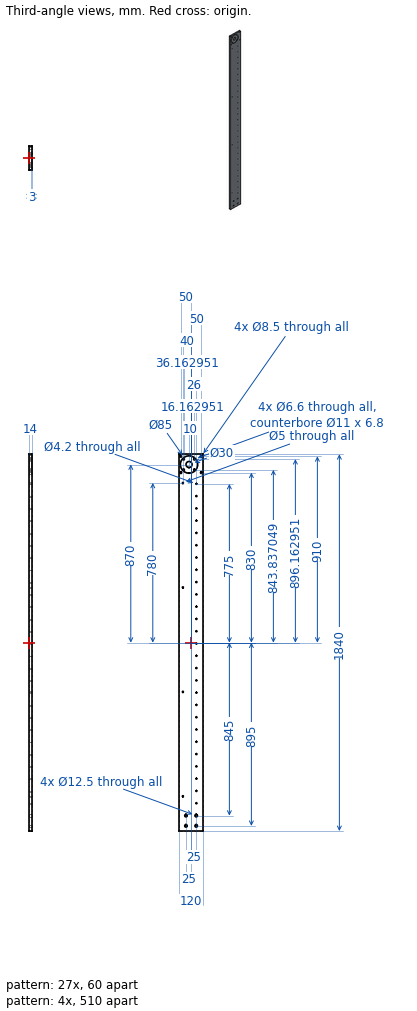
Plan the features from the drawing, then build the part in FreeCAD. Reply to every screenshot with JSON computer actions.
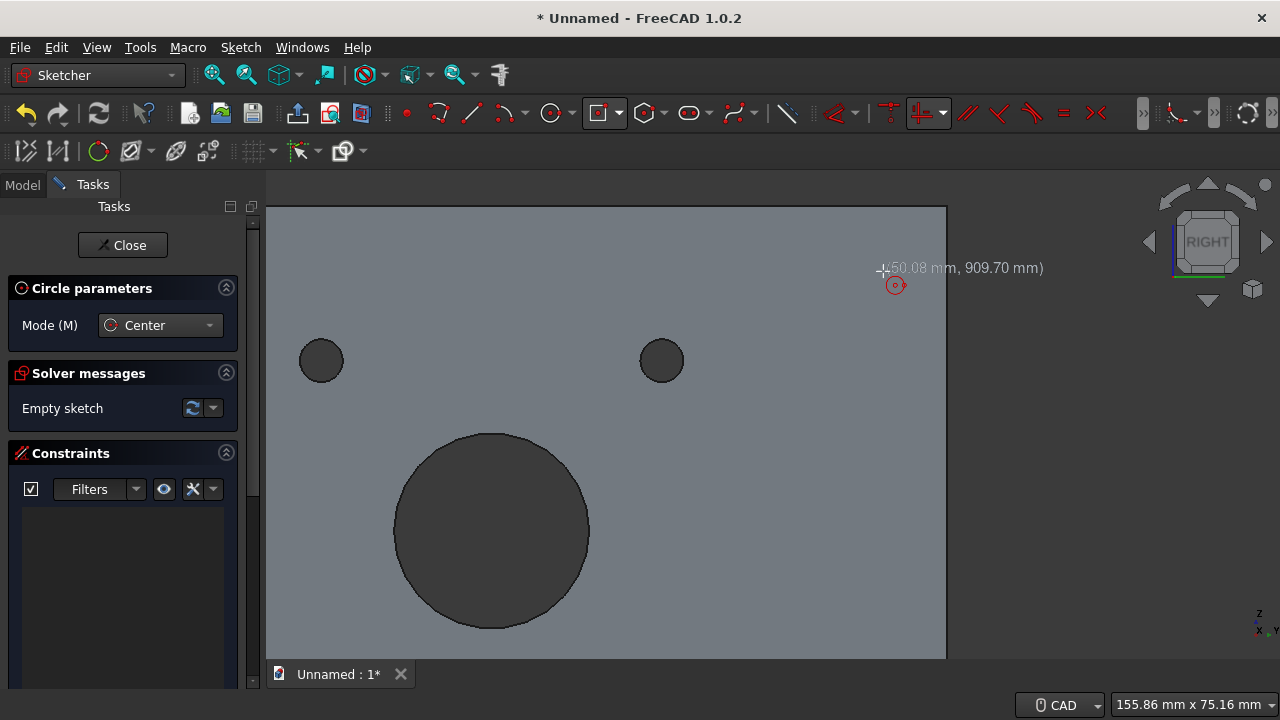
{"action": "left_click", "coordinate": [882, 271]}
{"action": "mouse_move", "coordinate": [902, 251]}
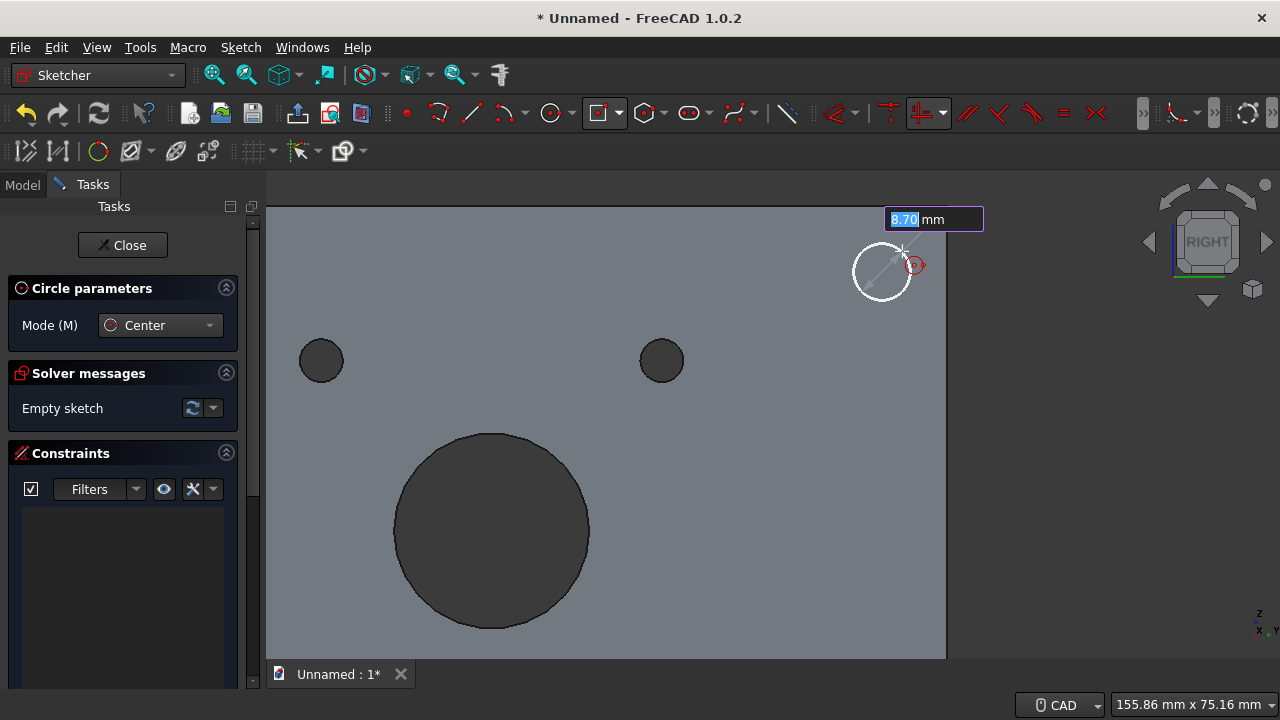
{"action": "type", "text": "8.5"}
{"action": "key", "text": "Return"}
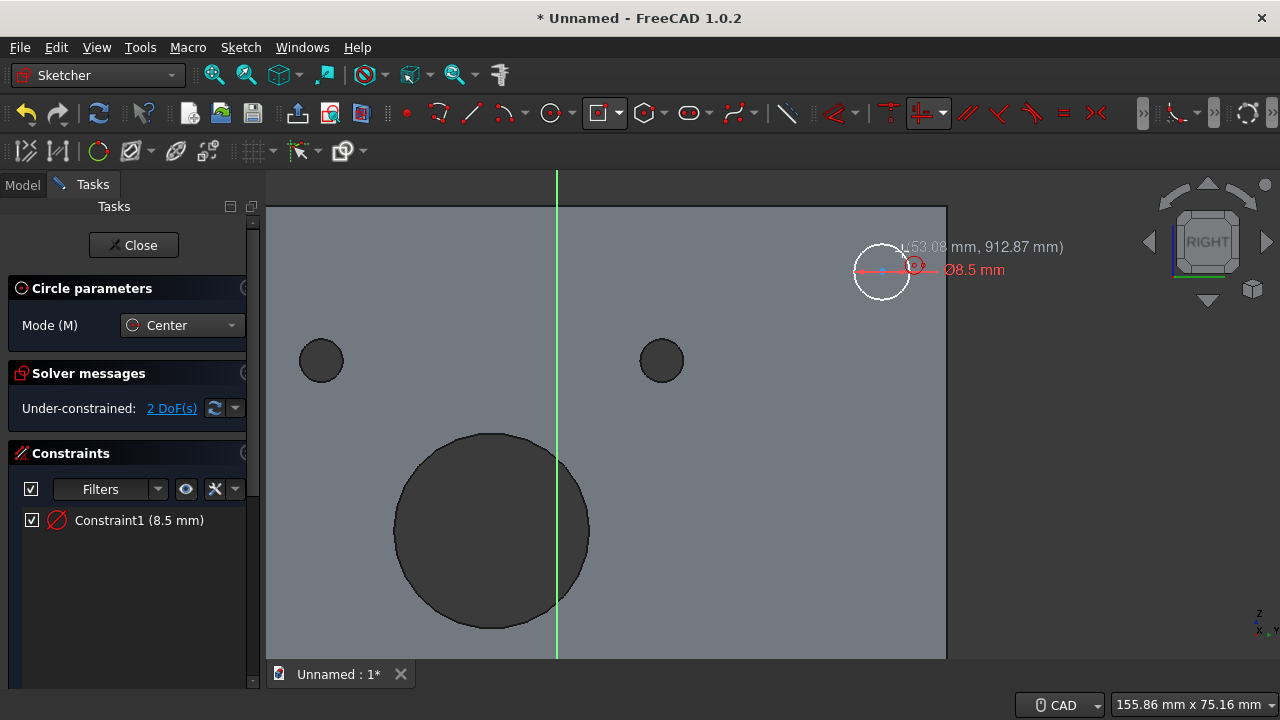
{"action": "scroll", "coordinate": [884, 273], "scroll_direction": "down", "scroll_amount": 3}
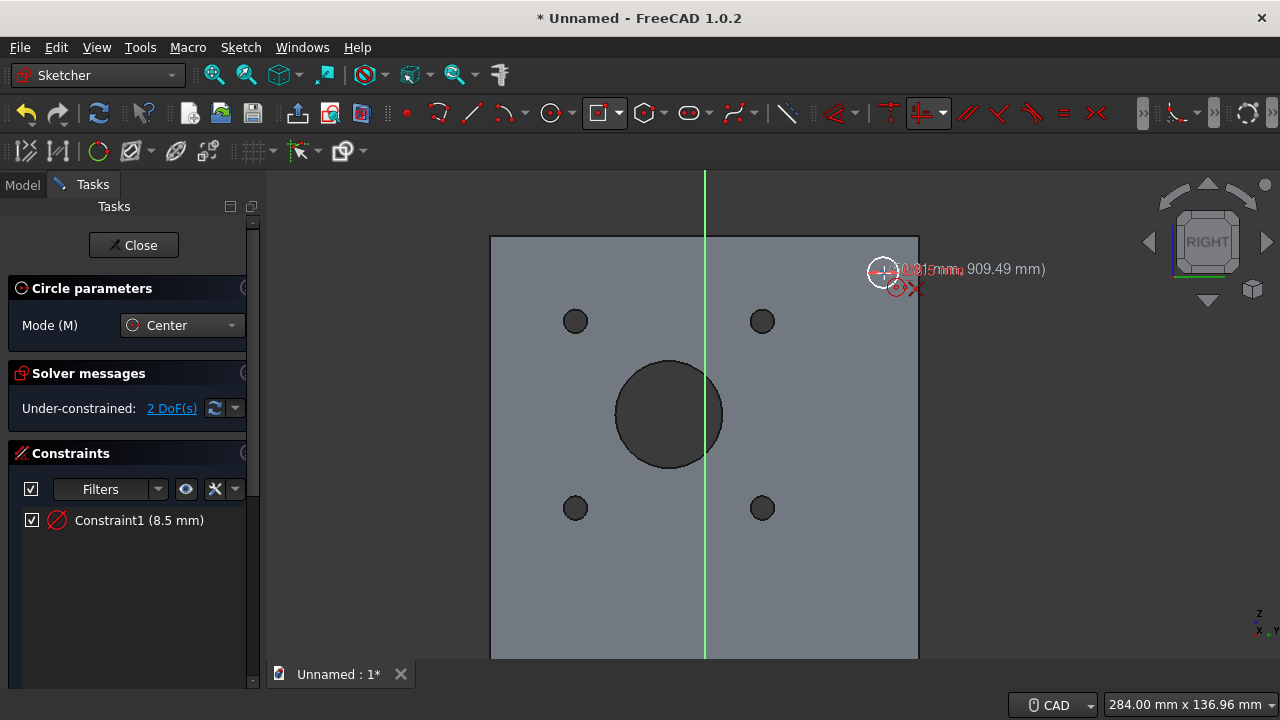
{"action": "scroll", "coordinate": [883, 557], "scroll_direction": "up", "scroll_amount": 3}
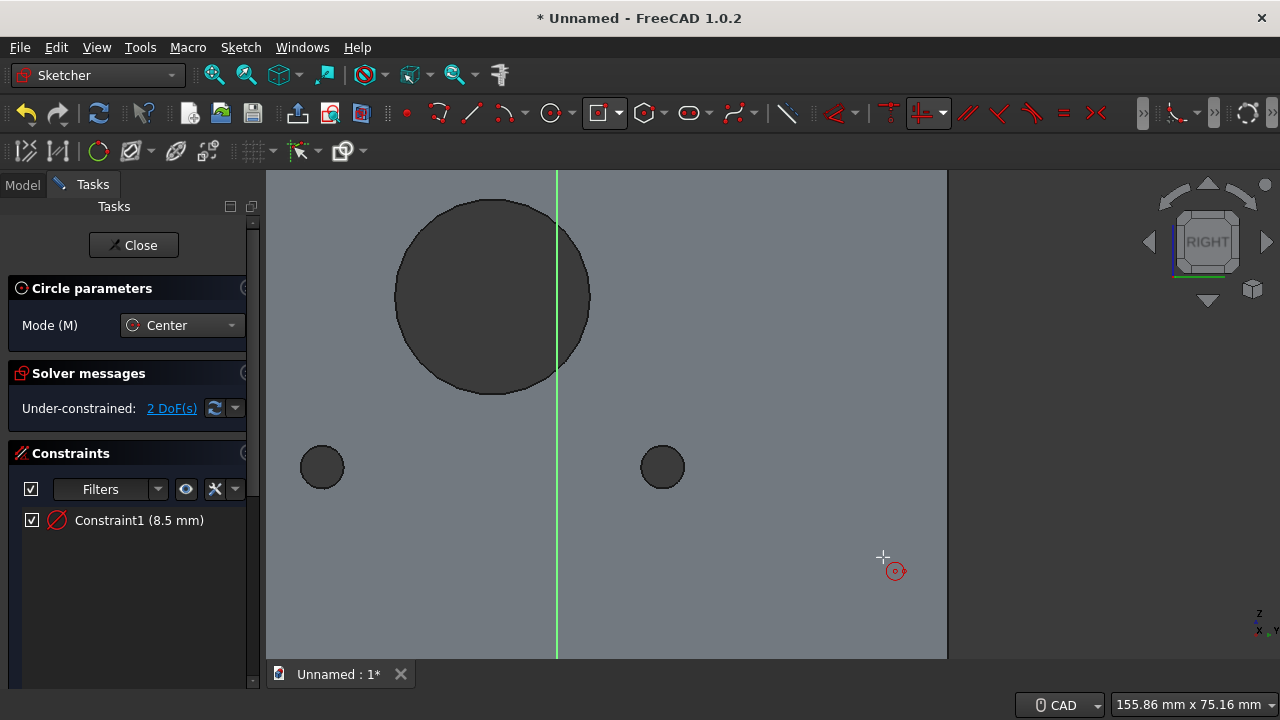
{"action": "left_click", "coordinate": [883, 557]}
{"action": "mouse_move", "coordinate": [902, 538]}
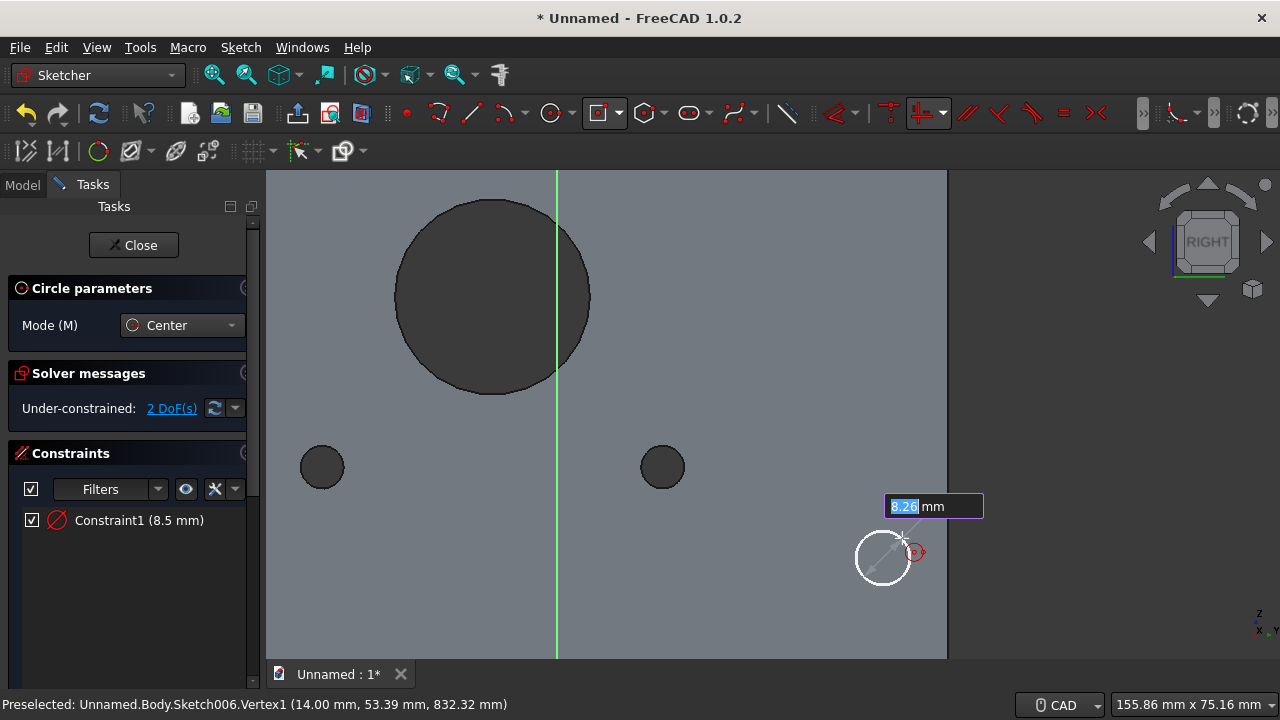
{"action": "type", "text": "8.5"}
{"action": "key", "text": "Return"}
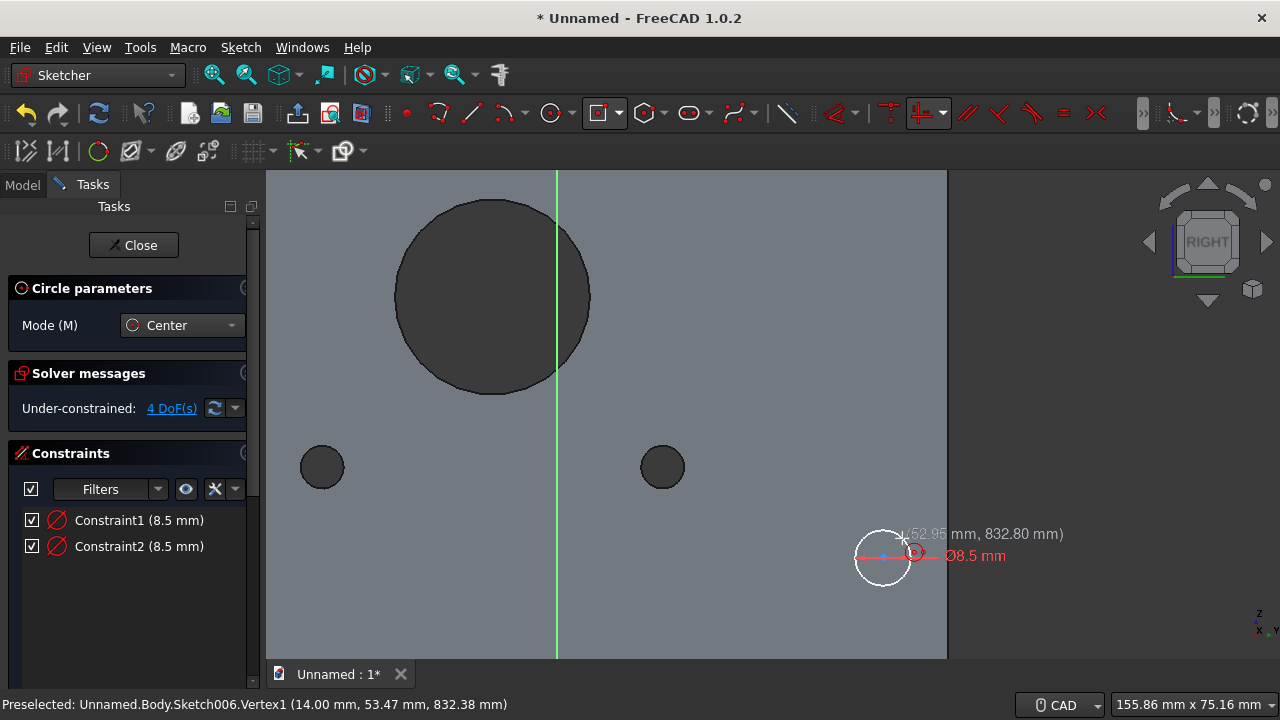
{"action": "scroll", "coordinate": [883, 557], "scroll_direction": "down", "scroll_amount": 3}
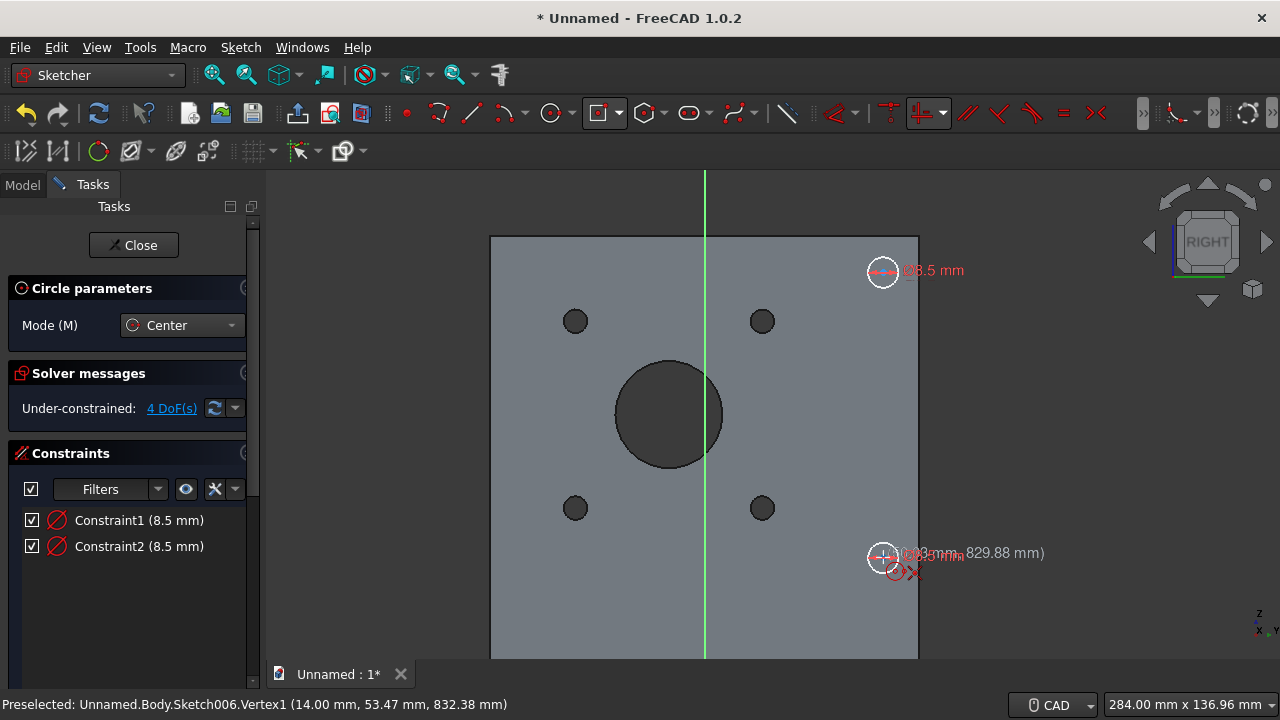
{"action": "scroll", "coordinate": [526, 272], "scroll_direction": "up", "scroll_amount": 3}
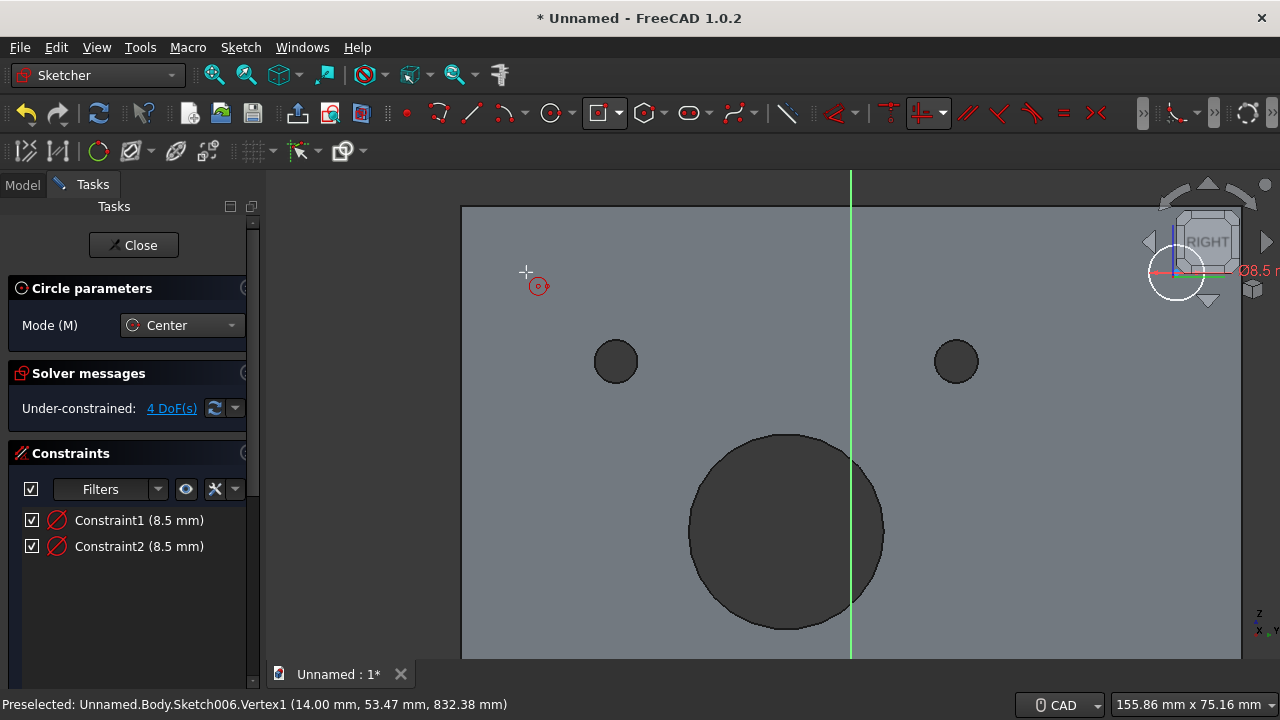
{"action": "left_click", "coordinate": [526, 272]}
{"action": "mouse_move", "coordinate": [546, 252]}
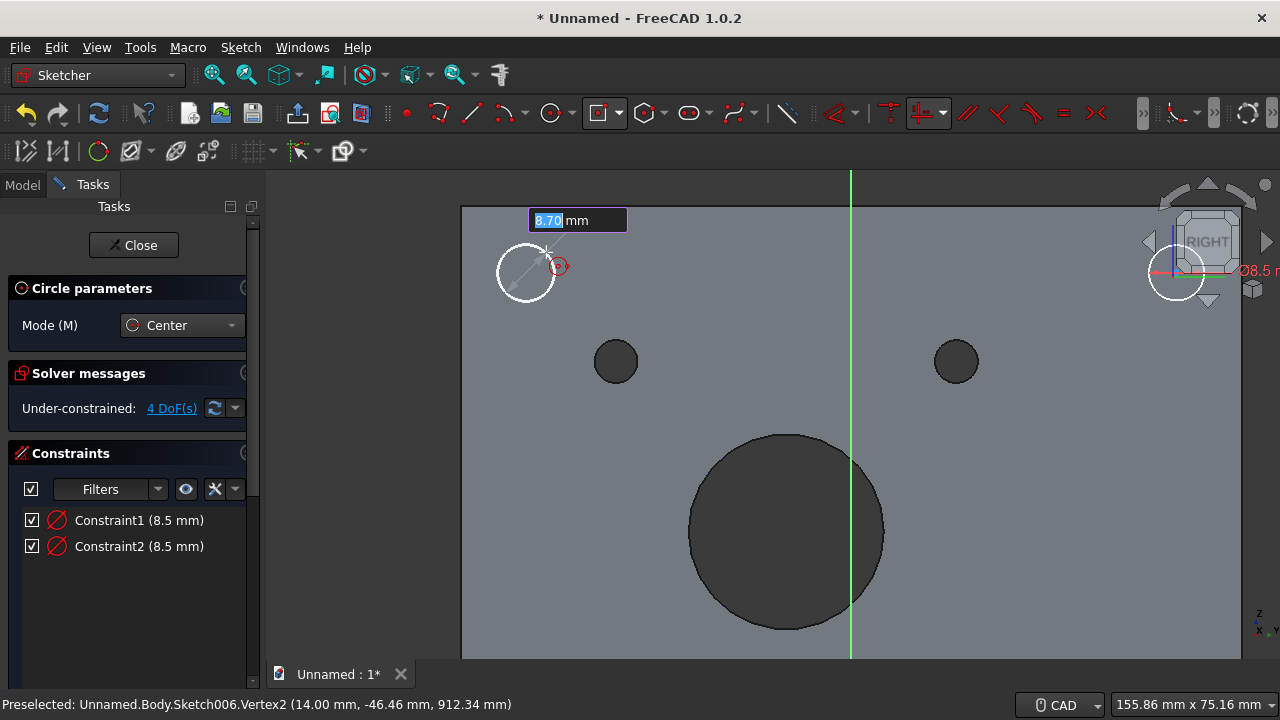
{"action": "type", "text": "8.5"}
{"action": "key", "text": "Return"}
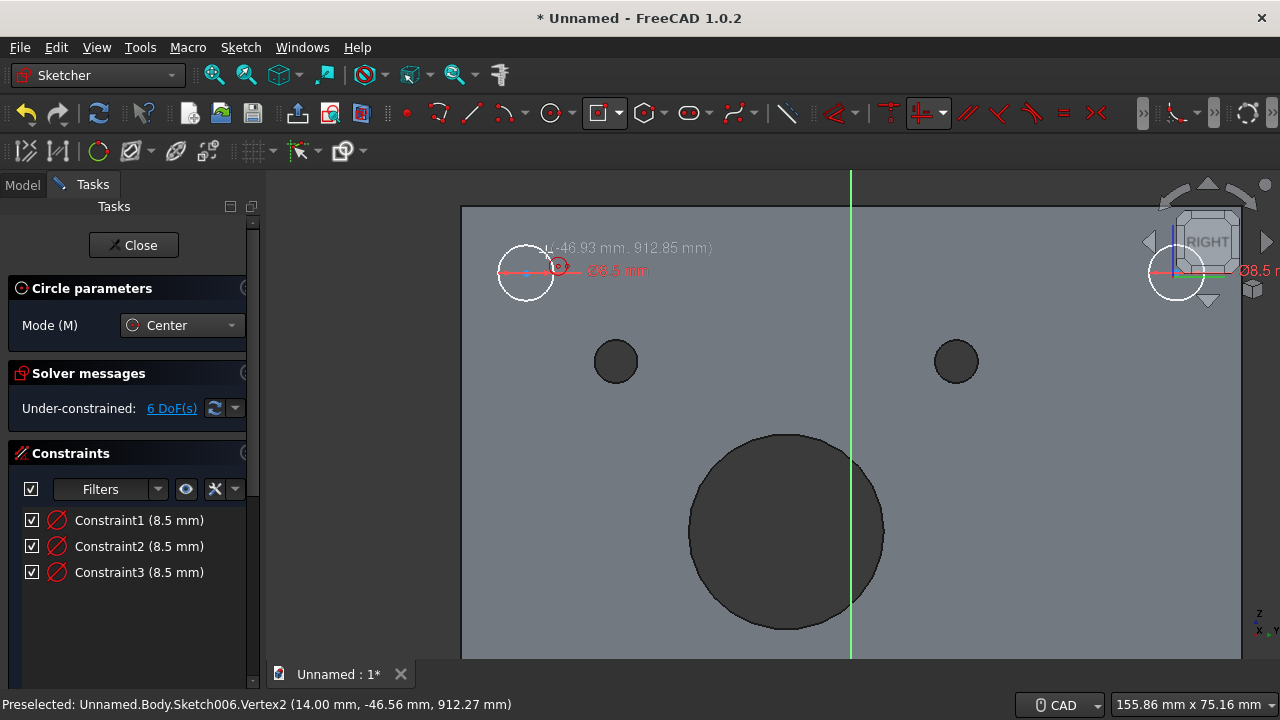
{"action": "scroll", "coordinate": [526, 272], "scroll_direction": "down", "scroll_amount": 3}